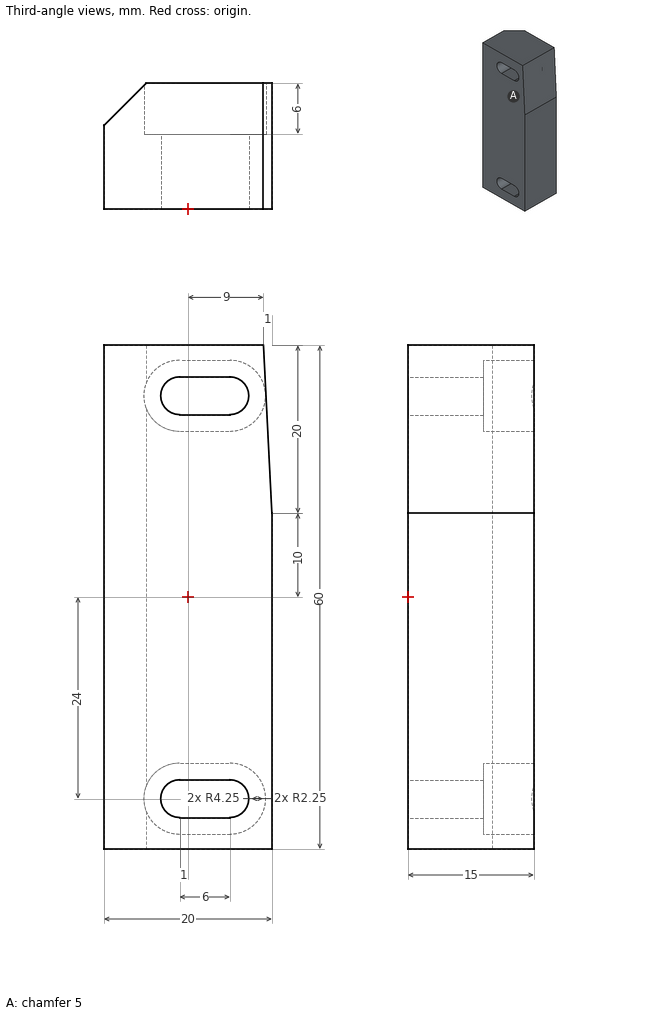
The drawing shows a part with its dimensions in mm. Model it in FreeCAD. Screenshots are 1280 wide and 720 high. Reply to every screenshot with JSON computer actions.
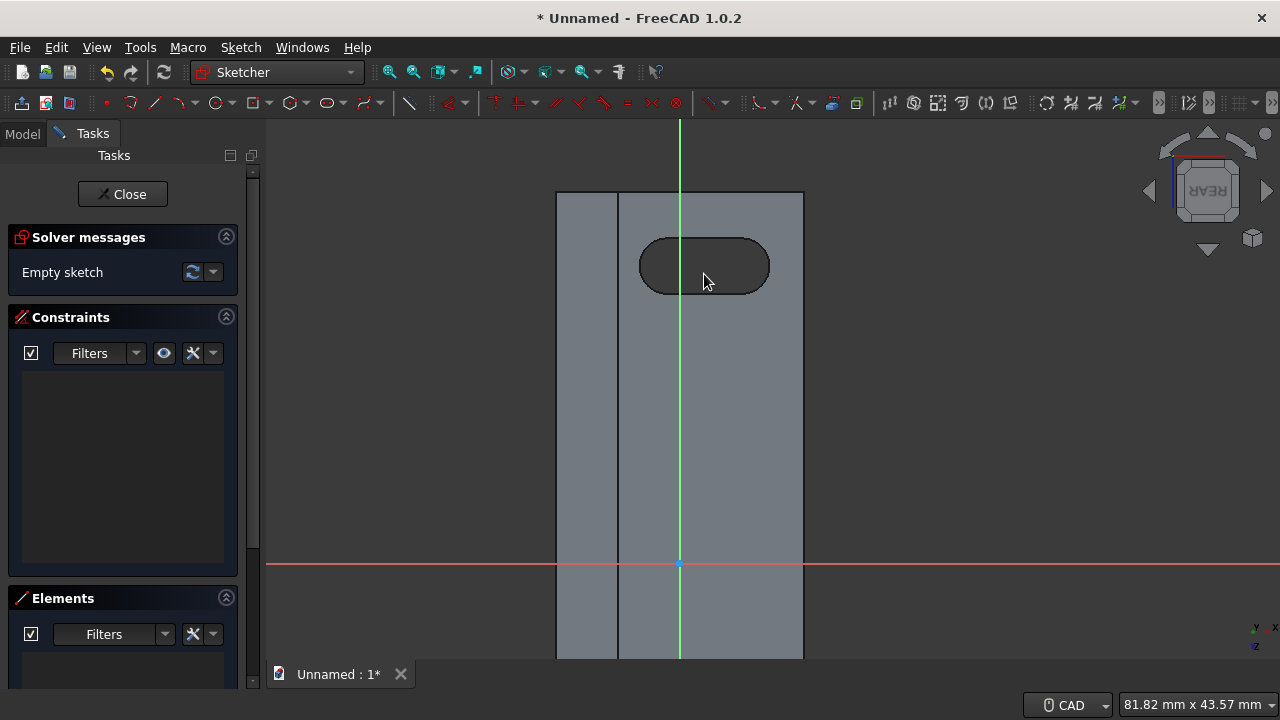
{"action": "left_click", "coordinate": [328, 104]}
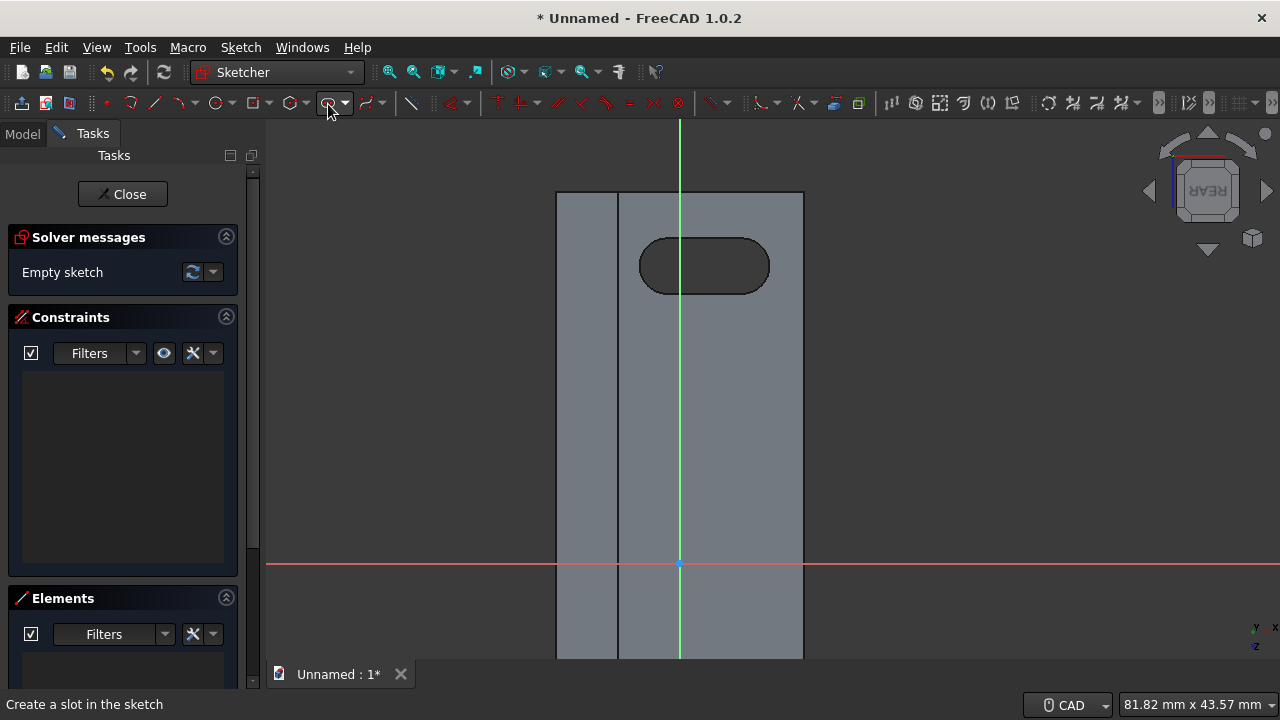
{"action": "scroll", "coordinate": [667, 266], "scroll_direction": "up", "scroll_amount": 2}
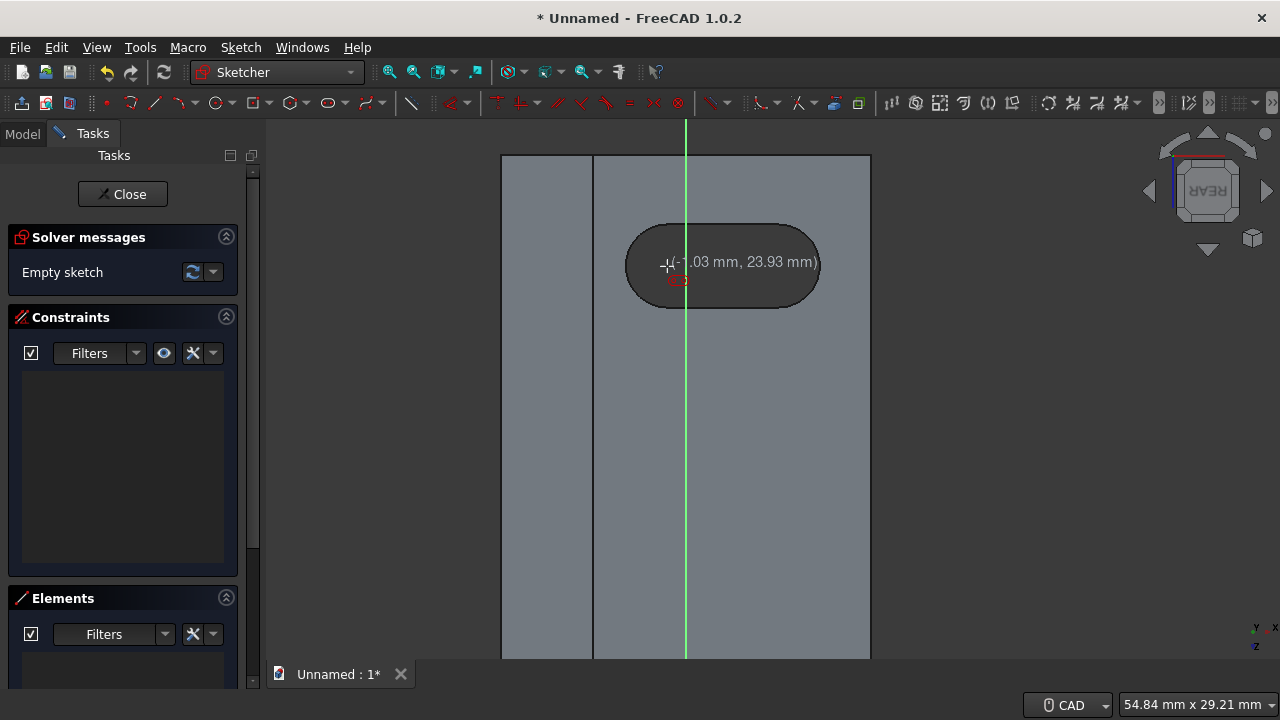
{"action": "left_click", "coordinate": [667, 266]}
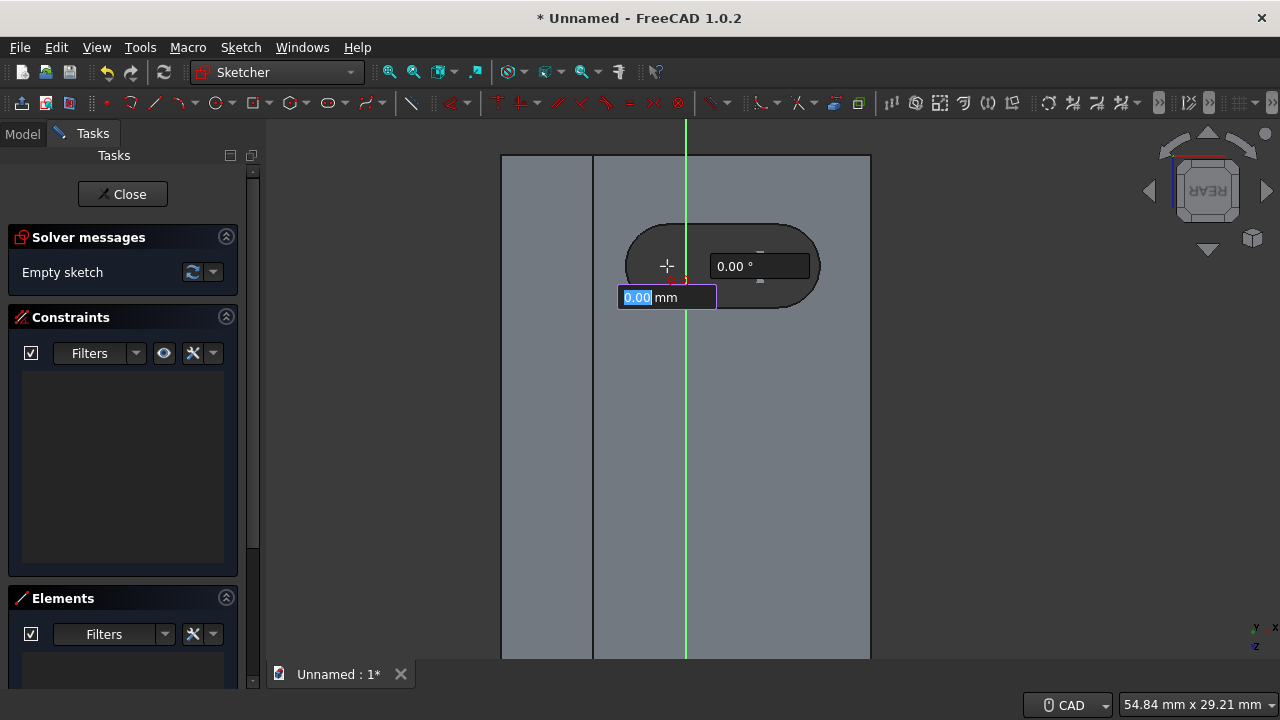
{"action": "left_click", "coordinate": [778, 266]}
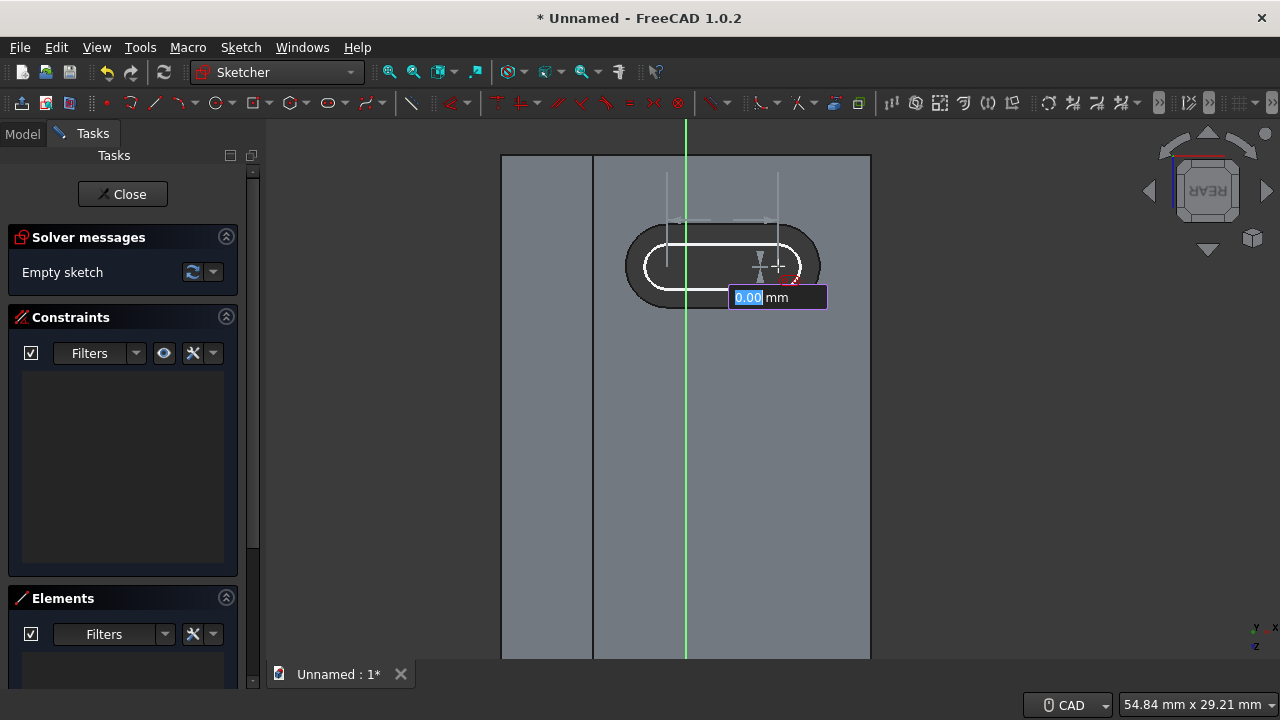
{"action": "left_click", "coordinate": [723, 345]}
{"action": "key", "text": "Escape"}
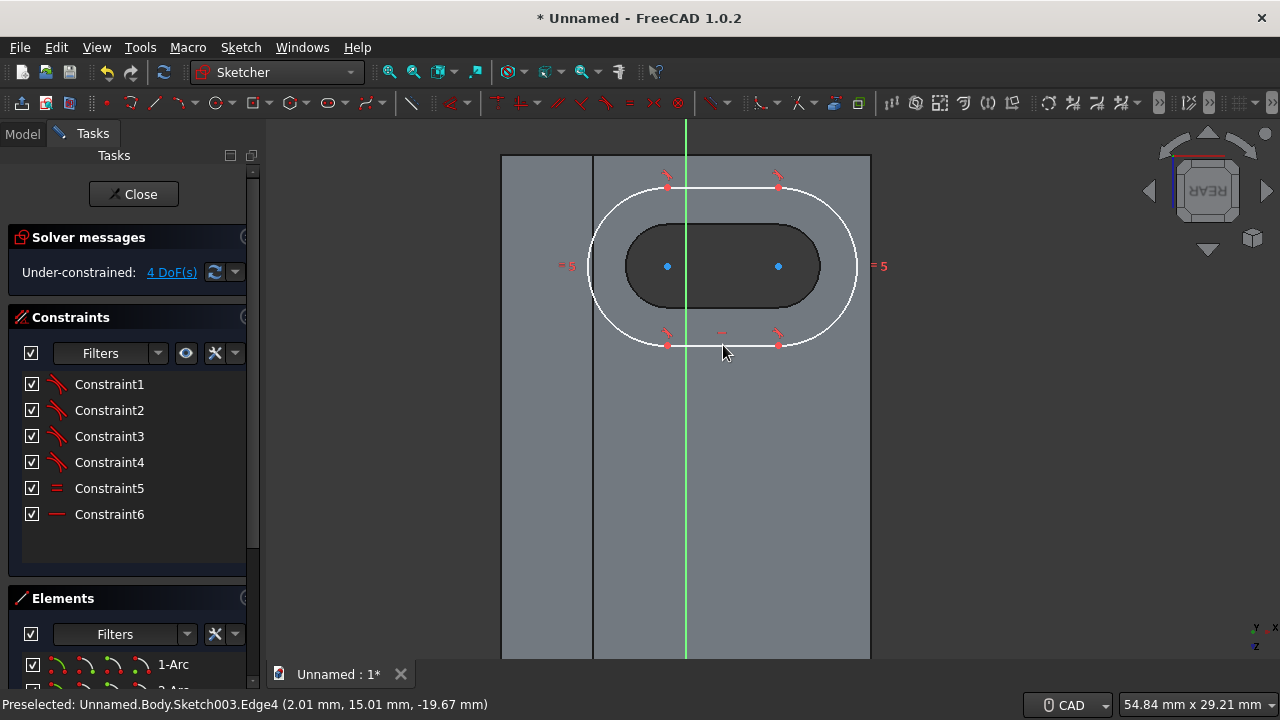
{"action": "left_click", "coordinate": [450, 104]}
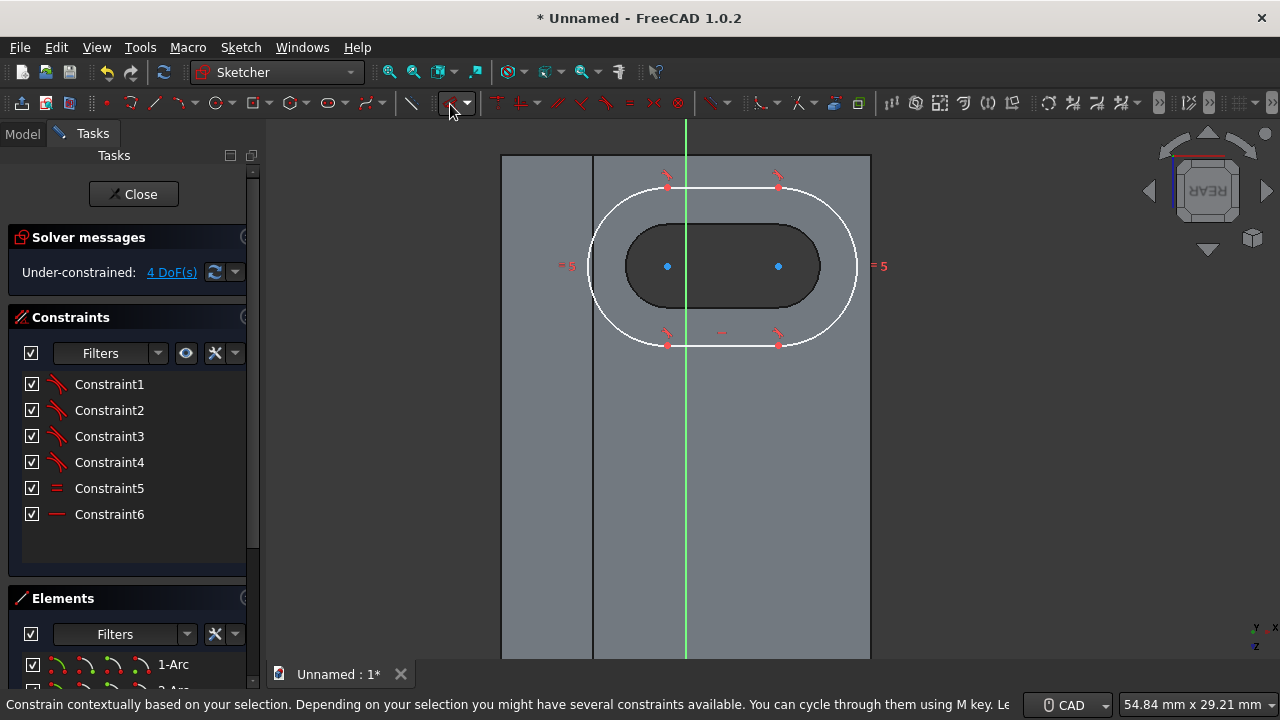
{"action": "left_click", "coordinate": [603, 221]}
{"action": "left_click", "coordinate": [577, 202]}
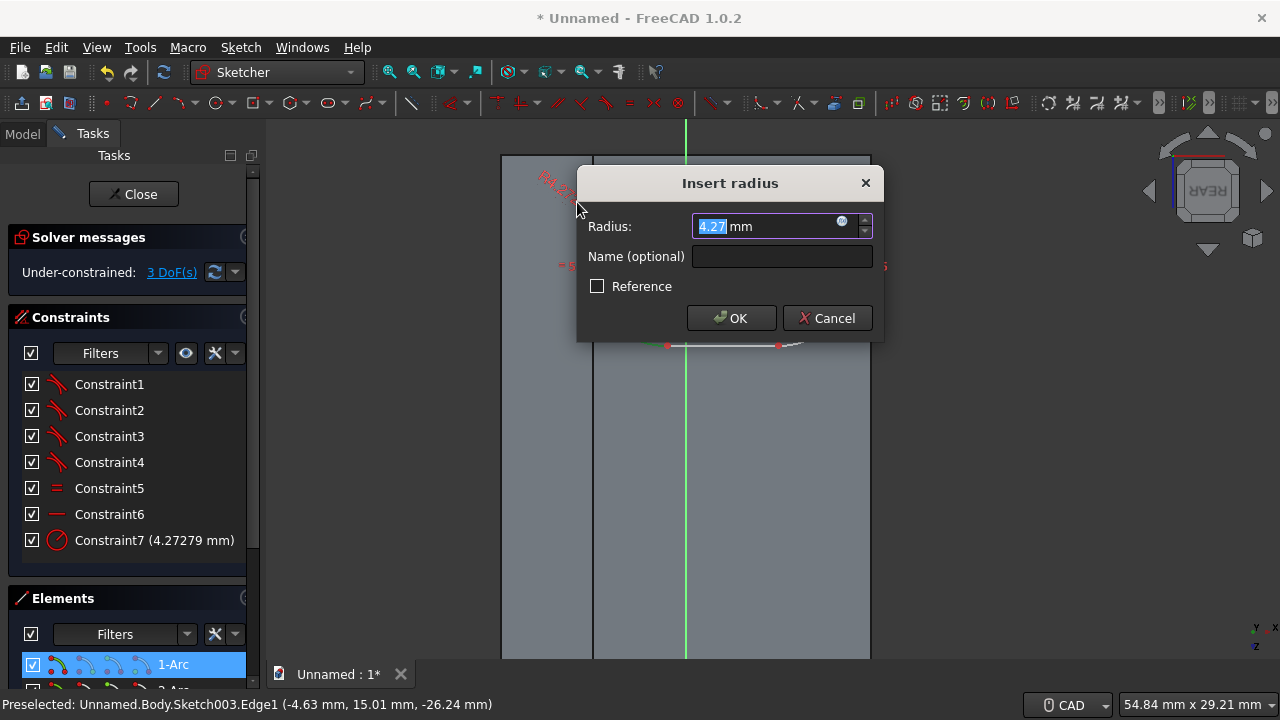
{"action": "type", "text": "4.25"}
{"action": "key", "text": "Return"}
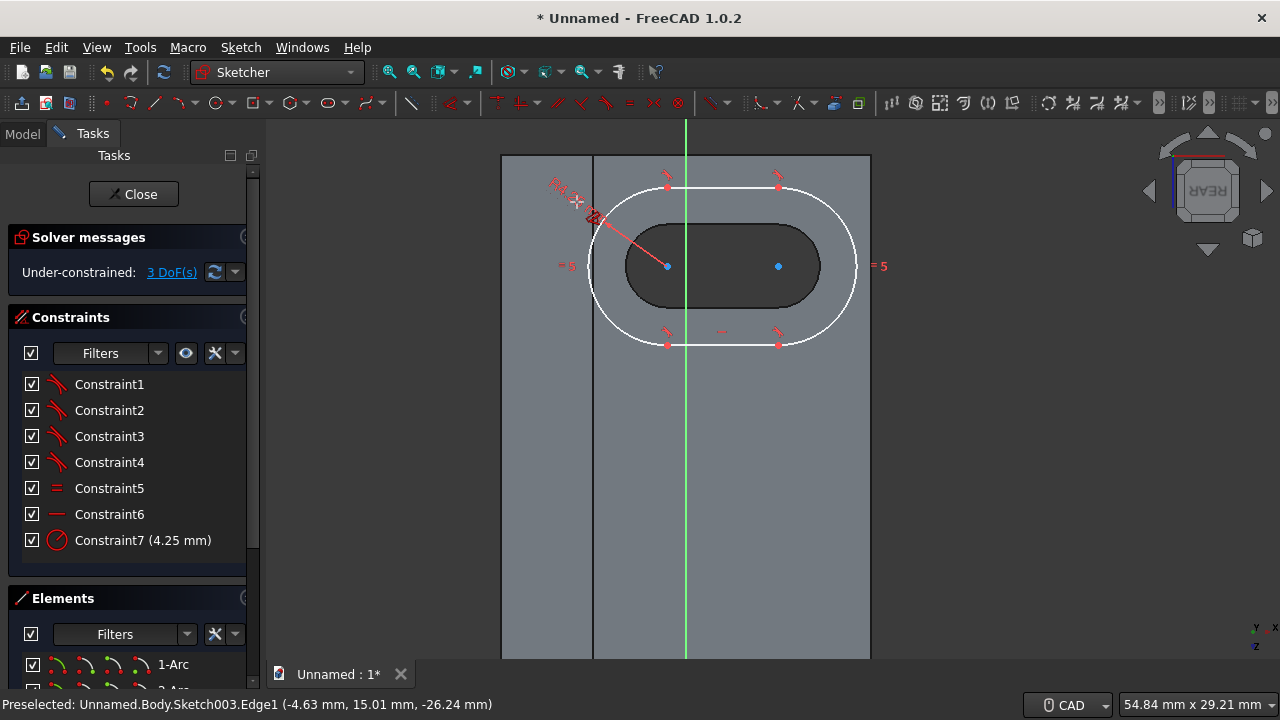
{"action": "left_click", "coordinate": [700, 188]}
{"action": "left_click", "coordinate": [722, 154]}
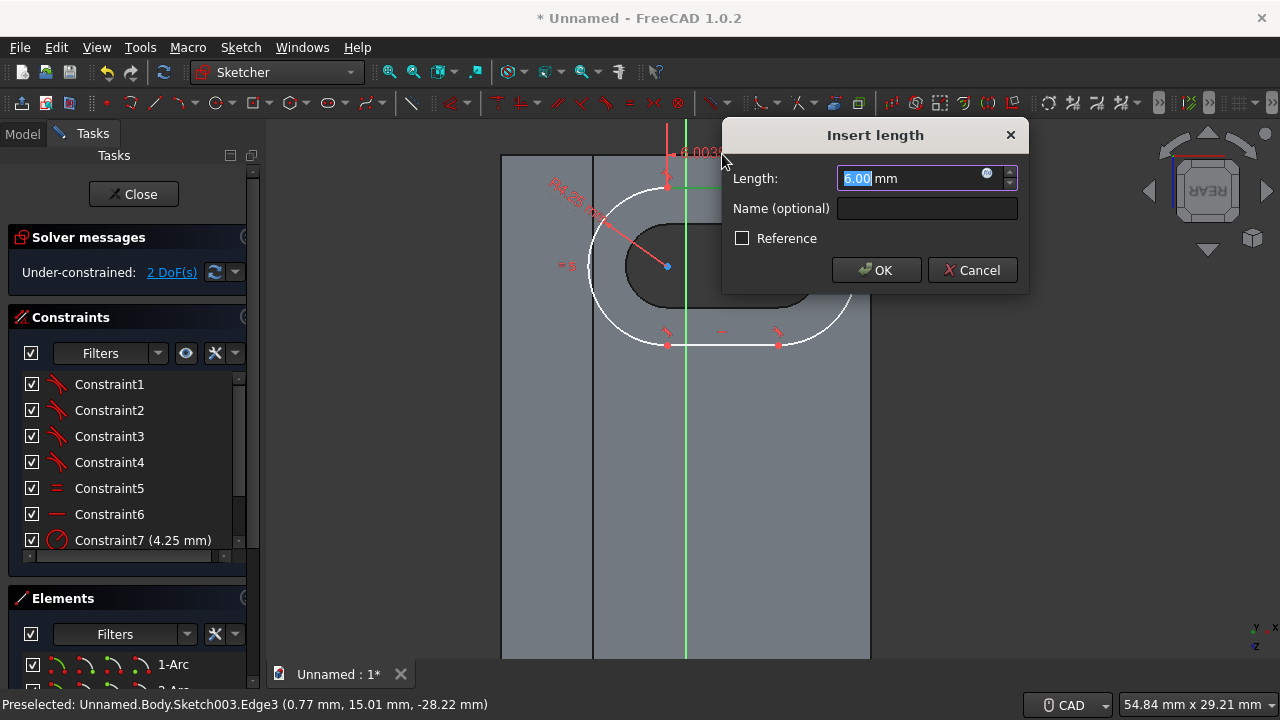
{"action": "type", "text": "6"}
{"action": "key", "text": "Return"}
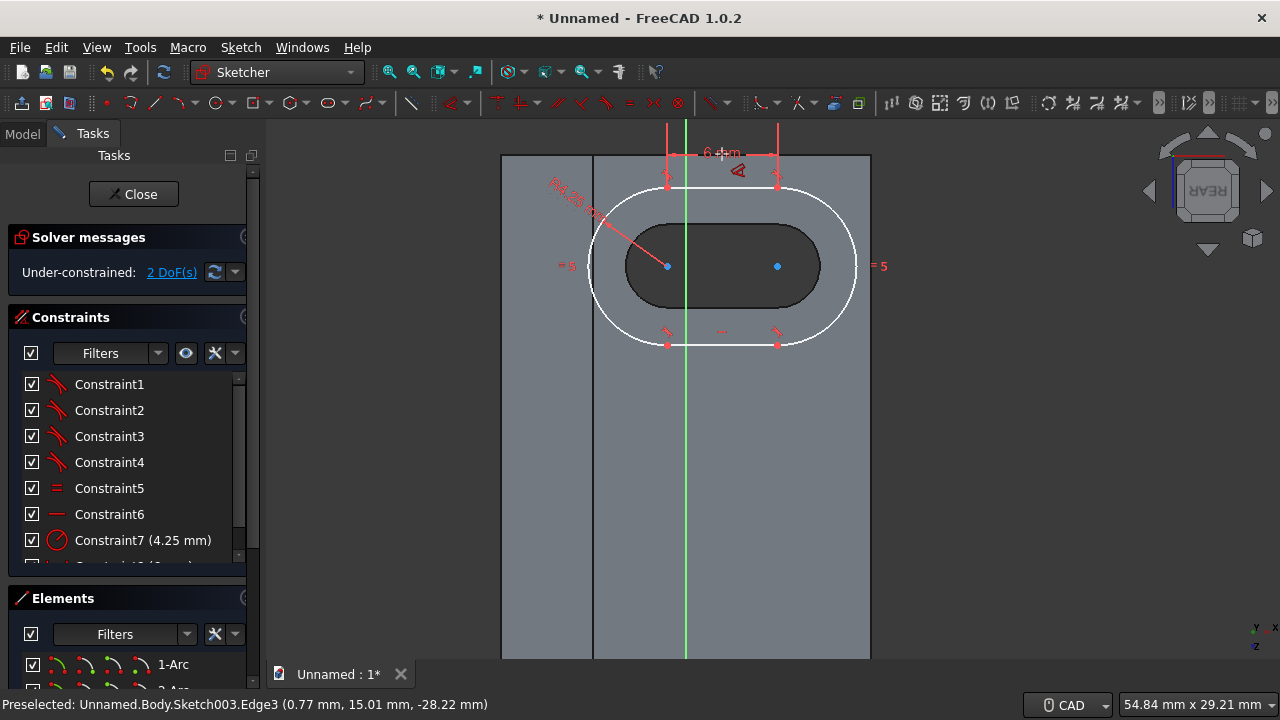
{"action": "scroll", "coordinate": [667, 188], "scroll_direction": "up", "scroll_amount": 4}